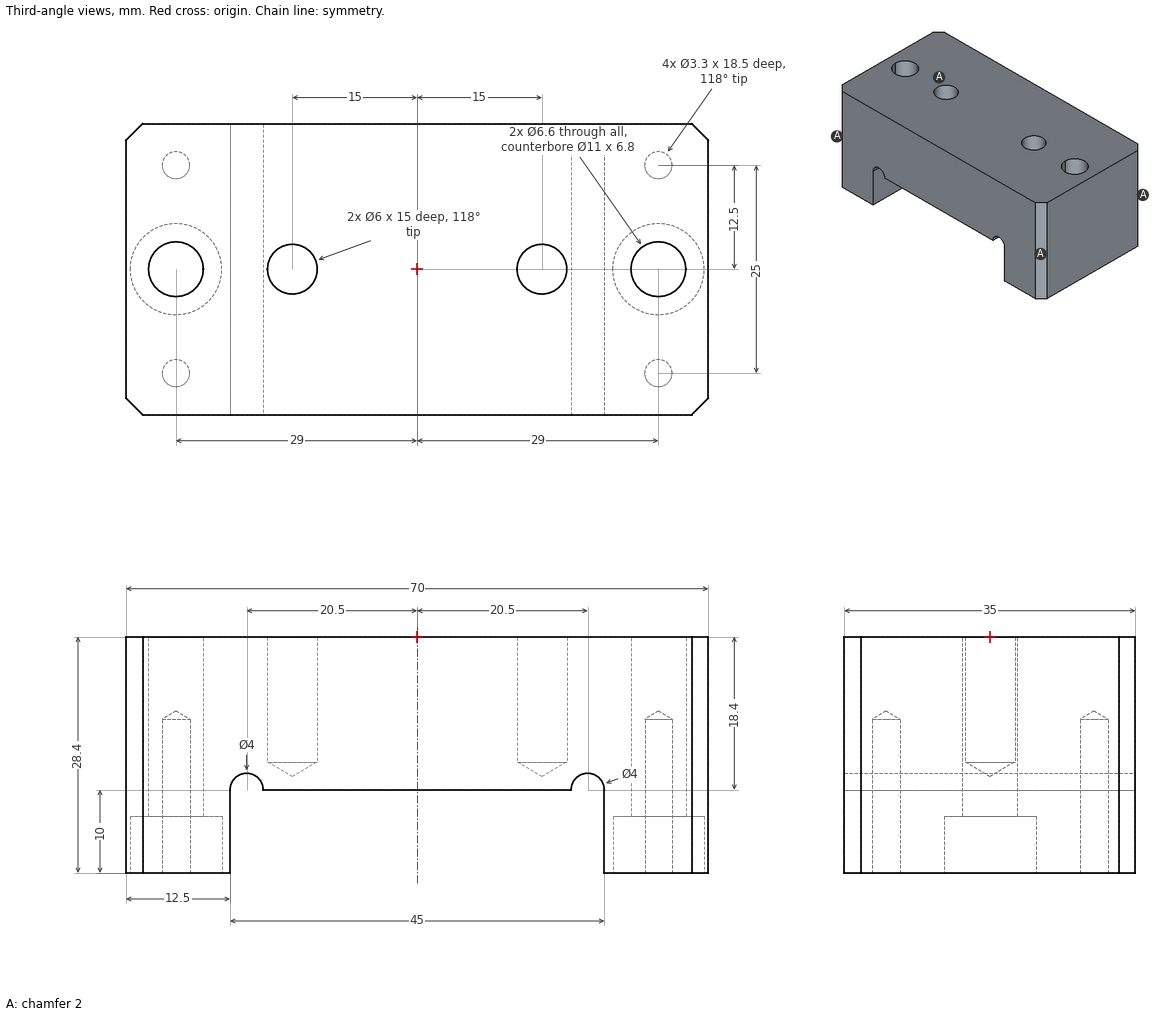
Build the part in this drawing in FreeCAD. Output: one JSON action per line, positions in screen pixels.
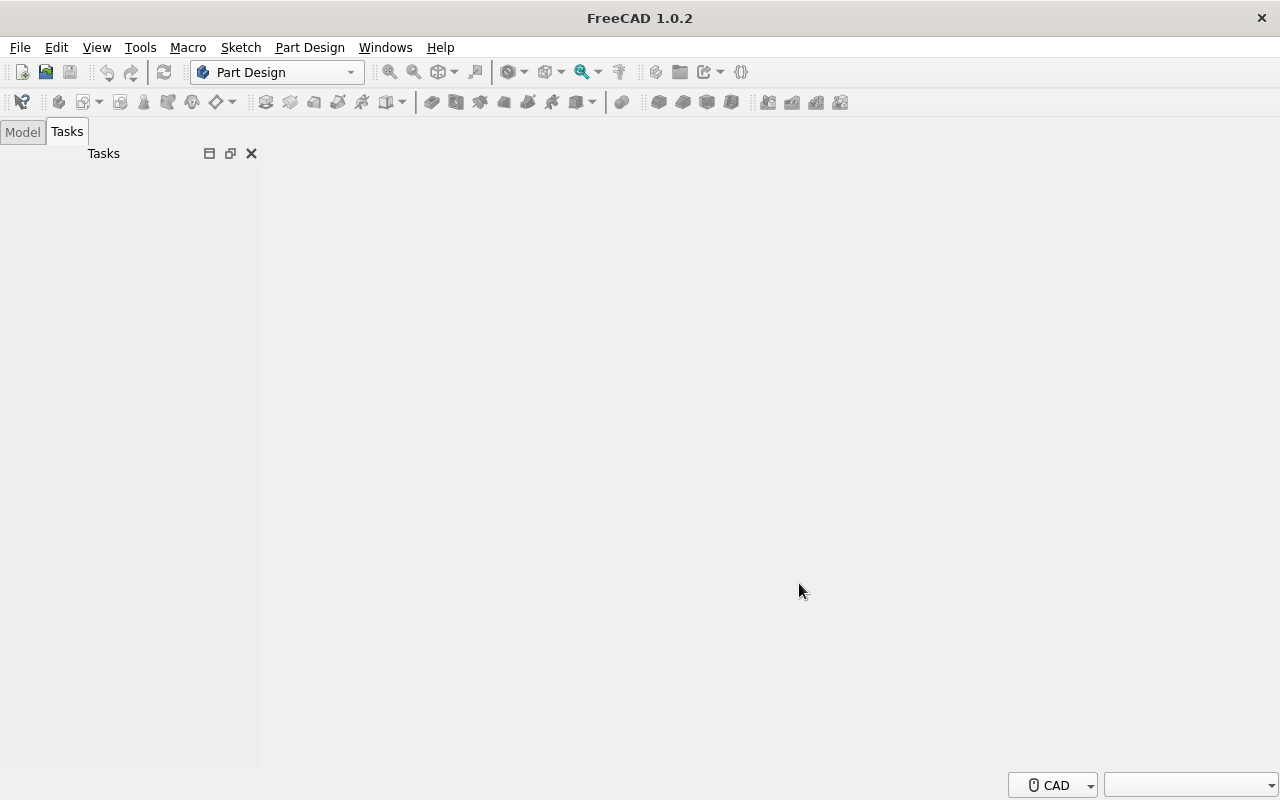
{"action": "left_click", "coordinate": [22, 72]}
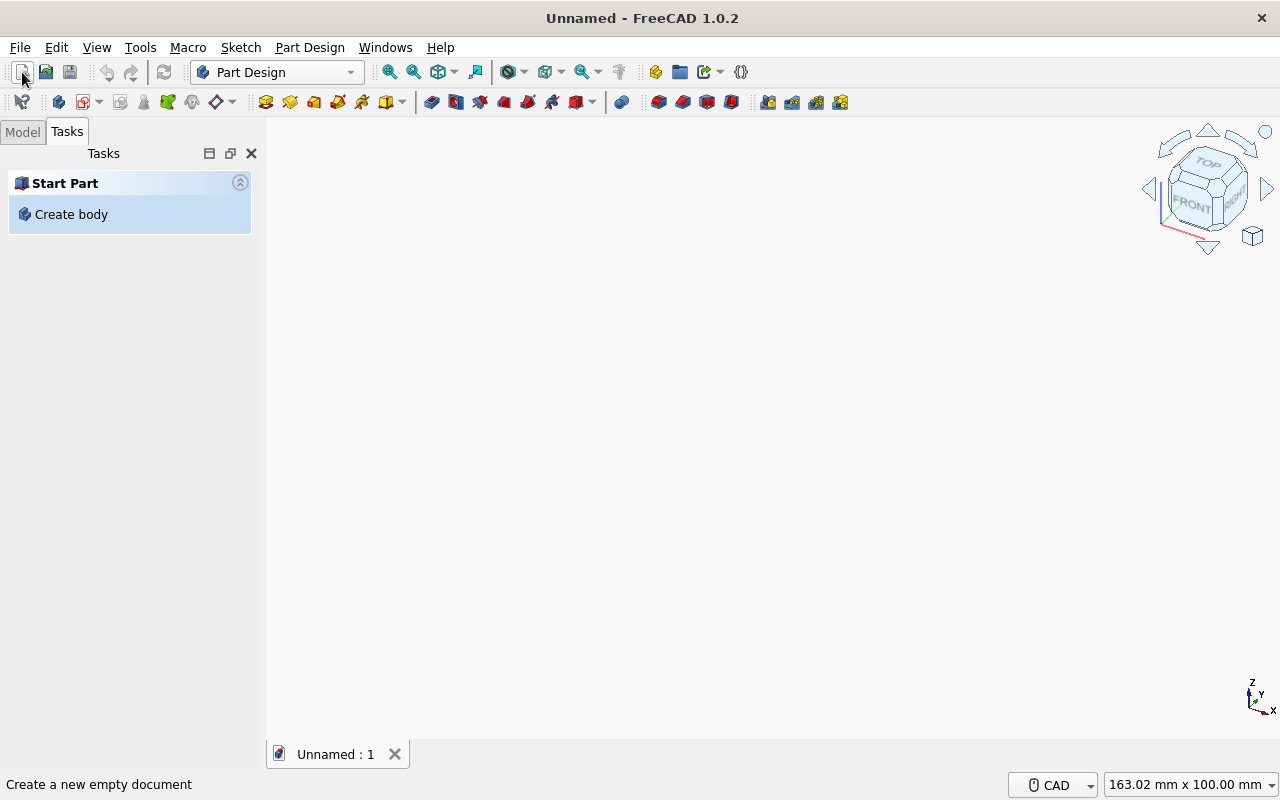
{"action": "left_click", "coordinate": [84, 102]}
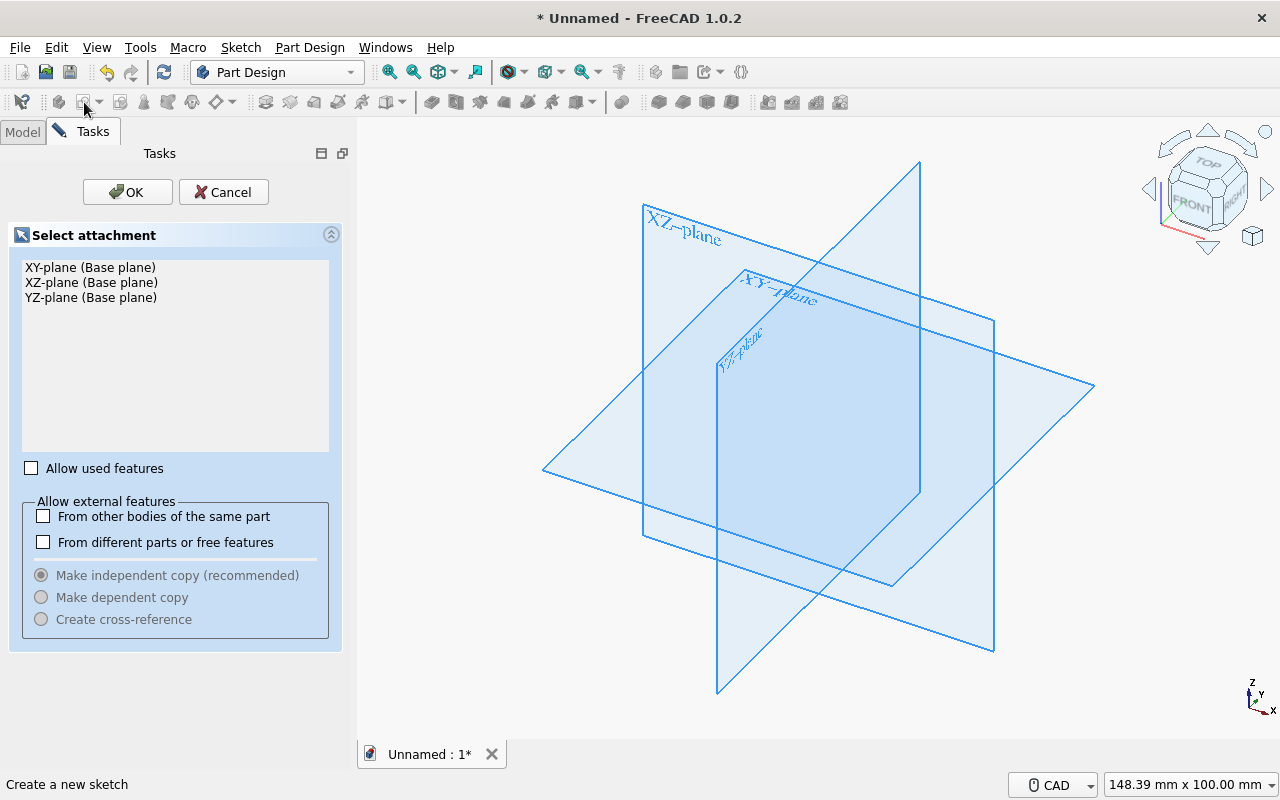
{"action": "left_click", "coordinate": [82, 282]}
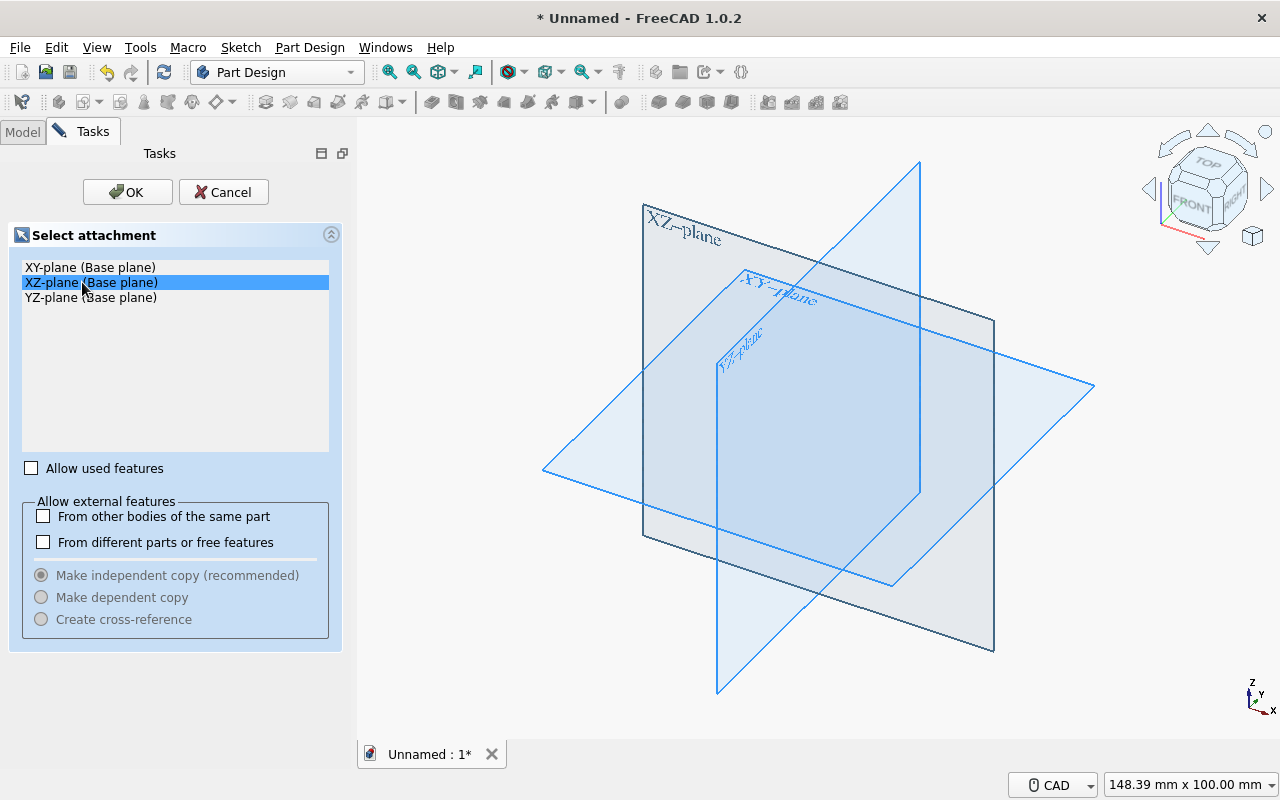
{"action": "left_click", "coordinate": [128, 192]}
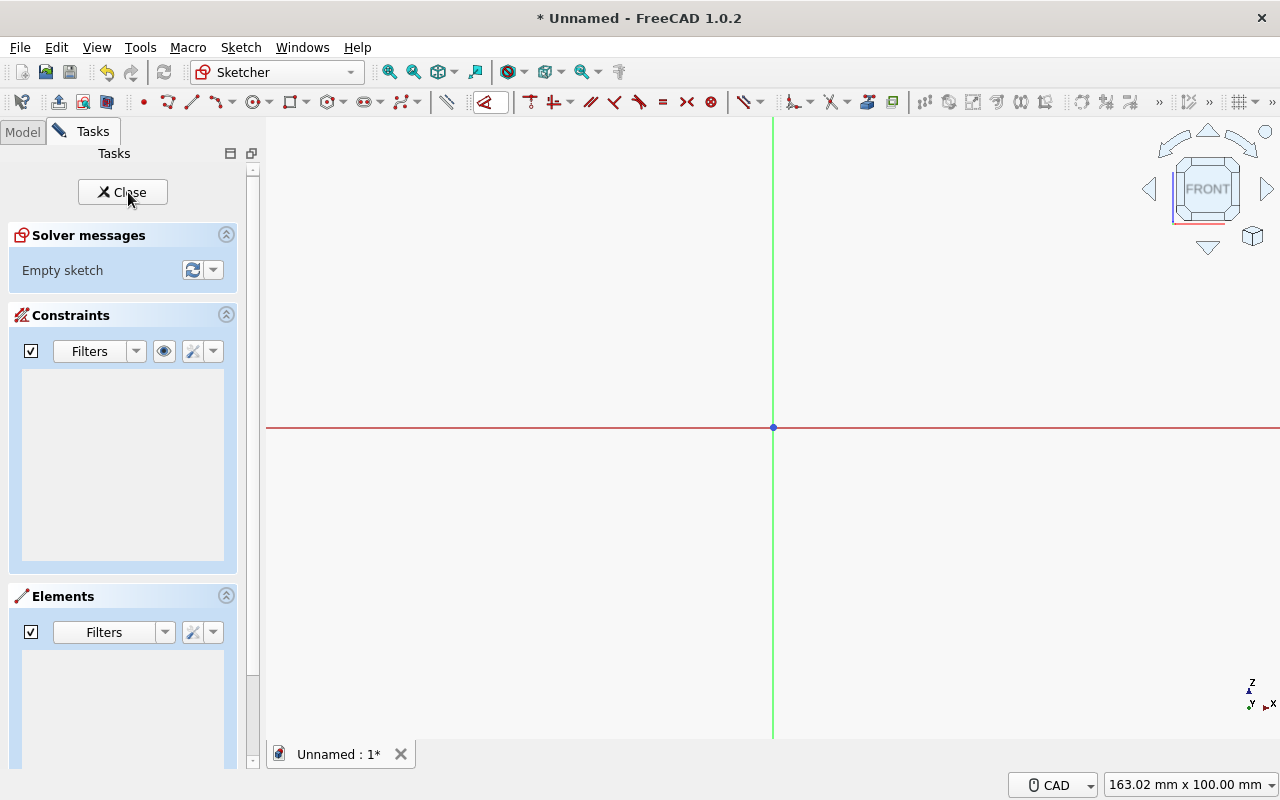
{"action": "key", "text": "g m"}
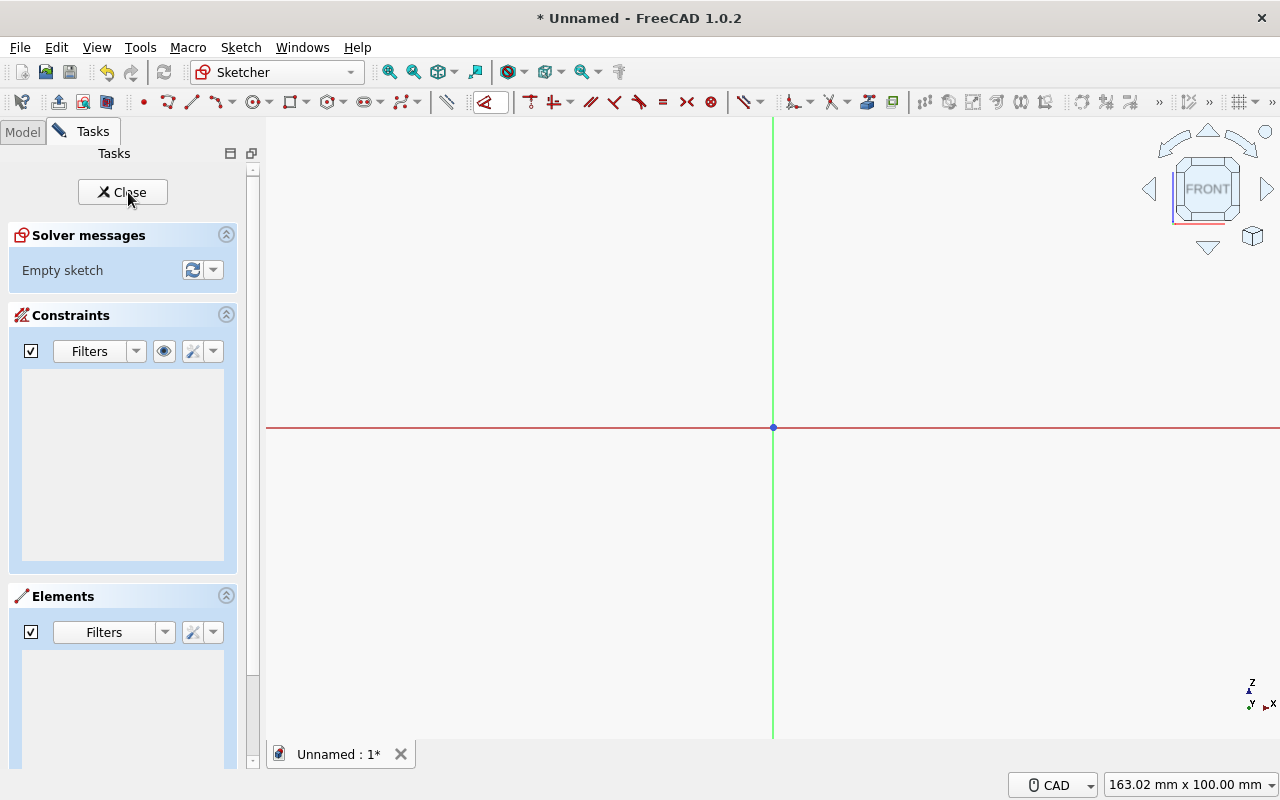
{"action": "left_click", "coordinate": [913, 542]}
{"action": "left_click", "coordinate": [633, 542]}
{"action": "left_click", "coordinate": [633, 605]}
{"action": "left_click", "coordinate": [555, 605]}
{"action": "left_click", "coordinate": [555, 428]}
{"action": "left_click", "coordinate": [991, 437]}
{"action": "left_click", "coordinate": [991, 605]}
{"action": "left_click", "coordinate": [913, 605]}
{"action": "left_click", "coordinate": [913, 543]}
{"action": "key", "text": "Escape"}
{"action": "key", "text": "Escape"}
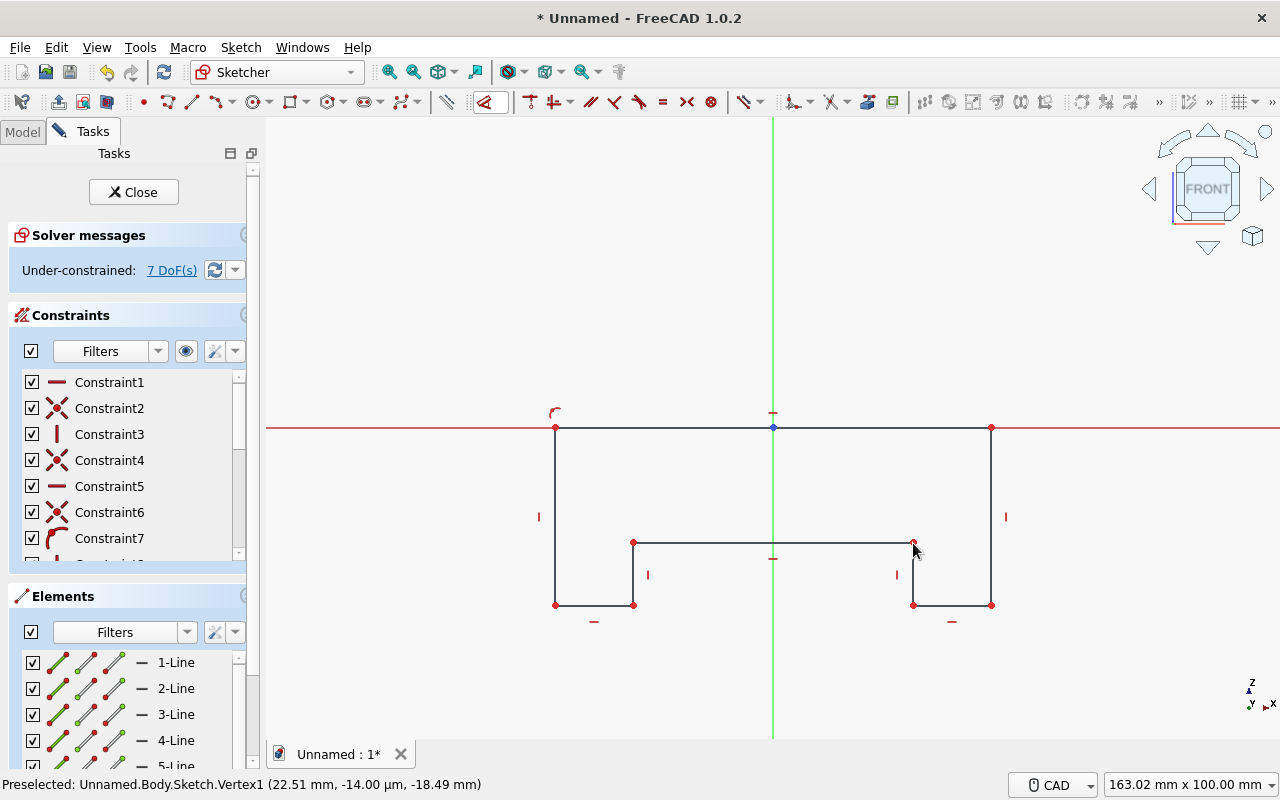
{"action": "left_click", "coordinate": [555, 606]}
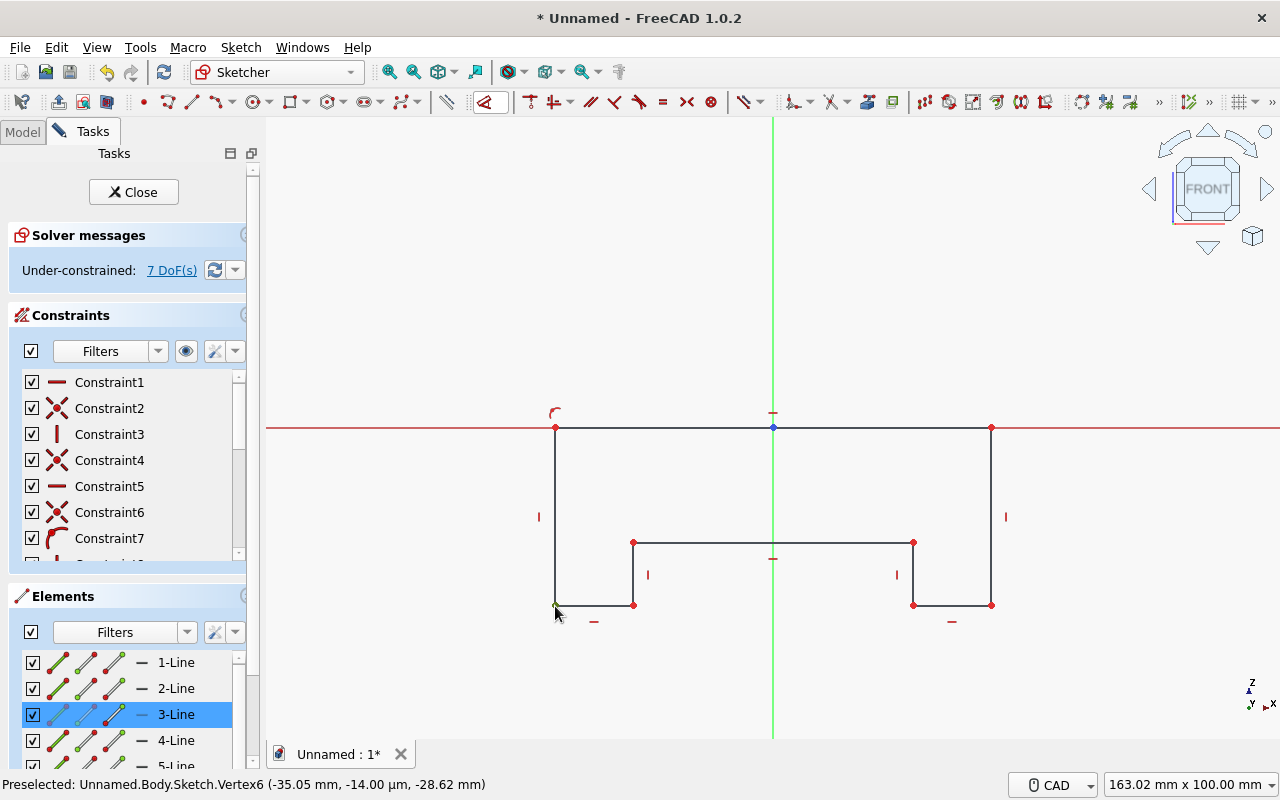
{"action": "left_click", "coordinate": [991, 606]}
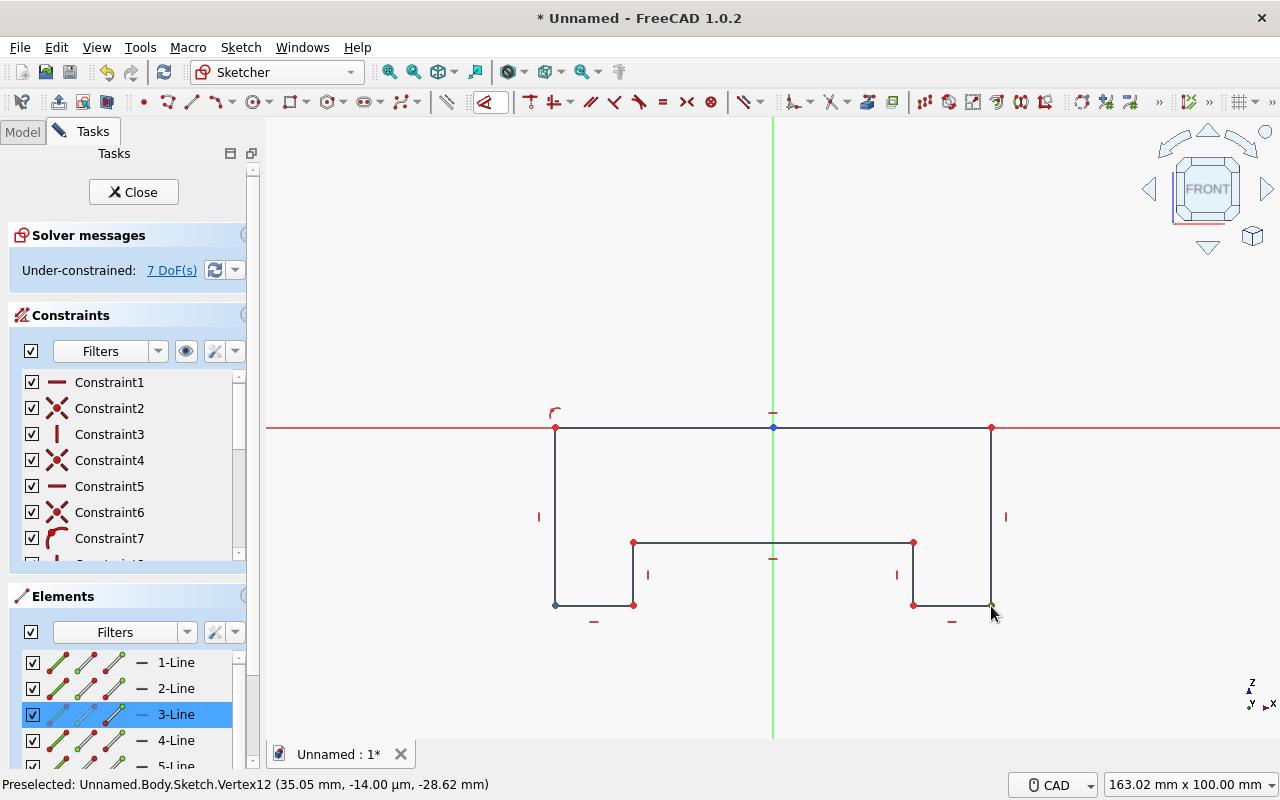
{"action": "left_click", "coordinate": [773, 671]}